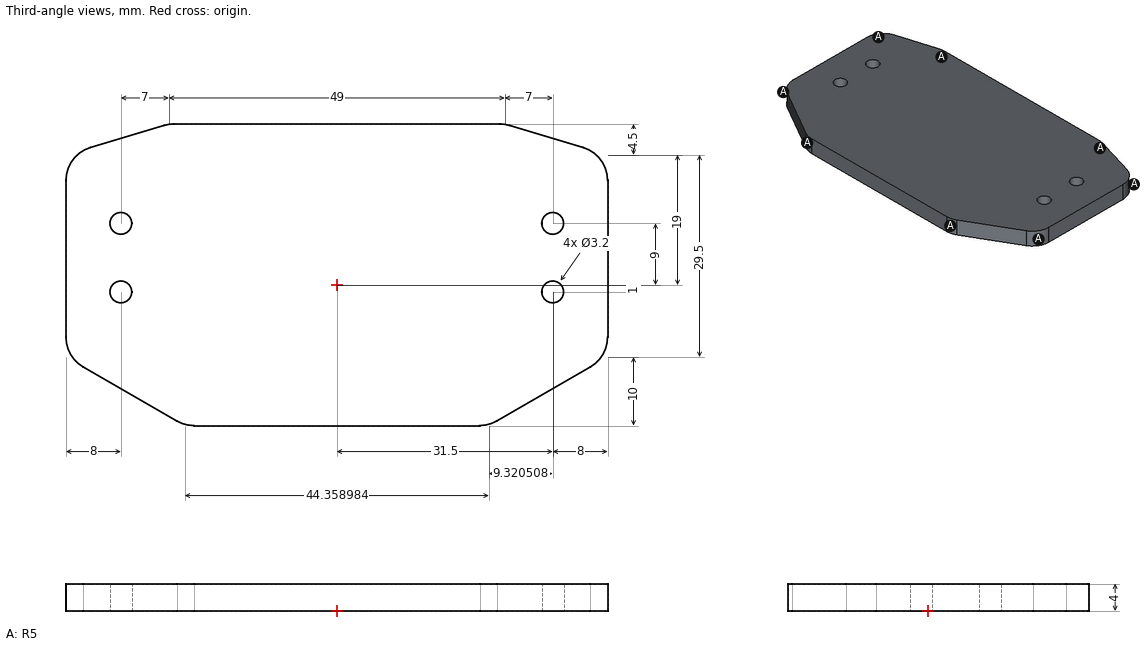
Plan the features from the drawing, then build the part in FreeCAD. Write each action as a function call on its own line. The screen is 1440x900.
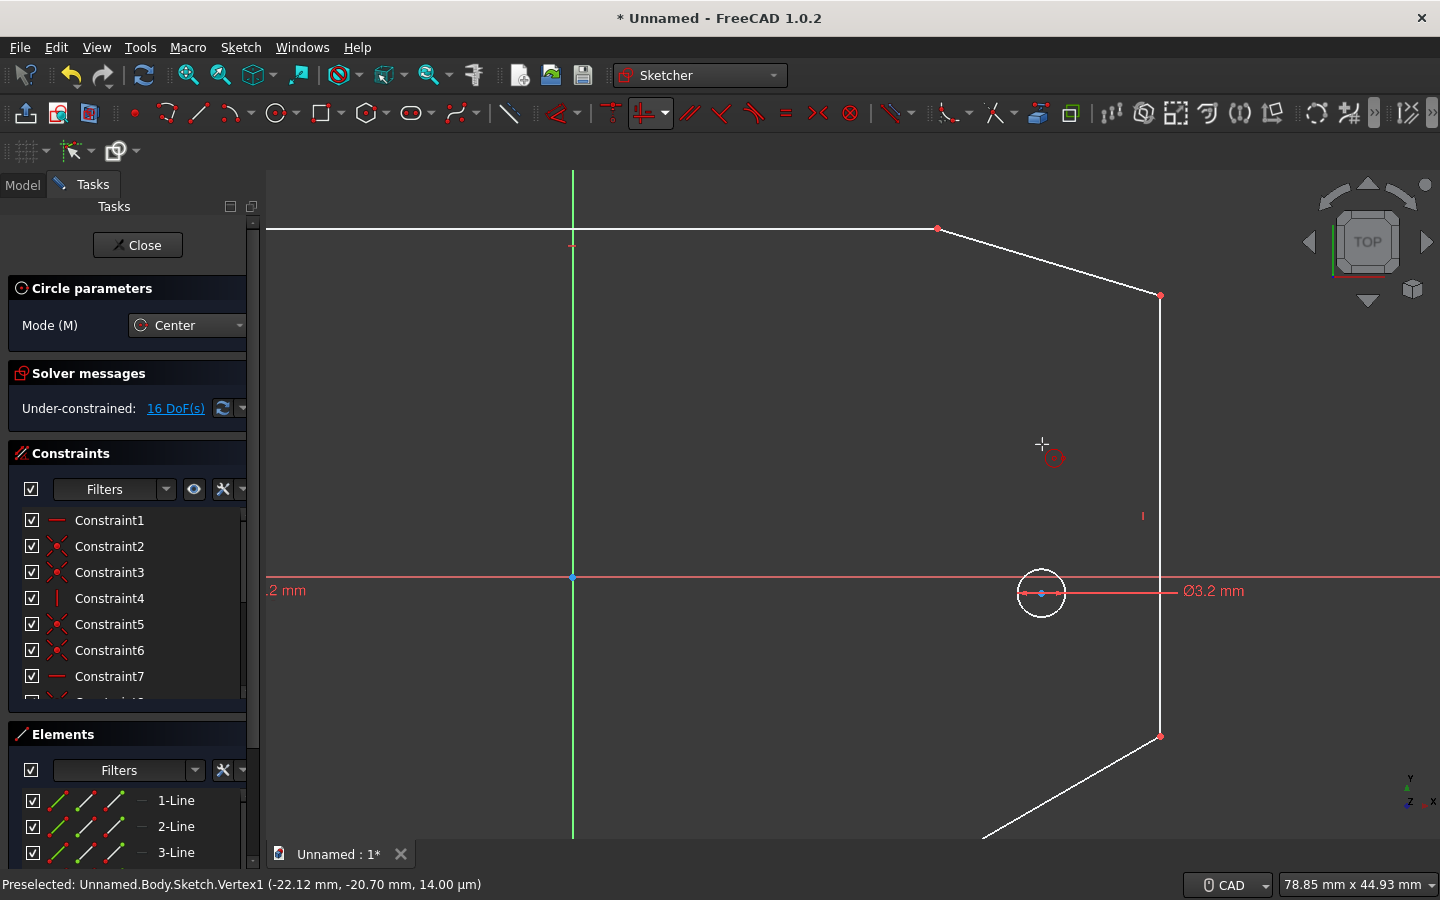
click(1042, 443)
move(1058, 426)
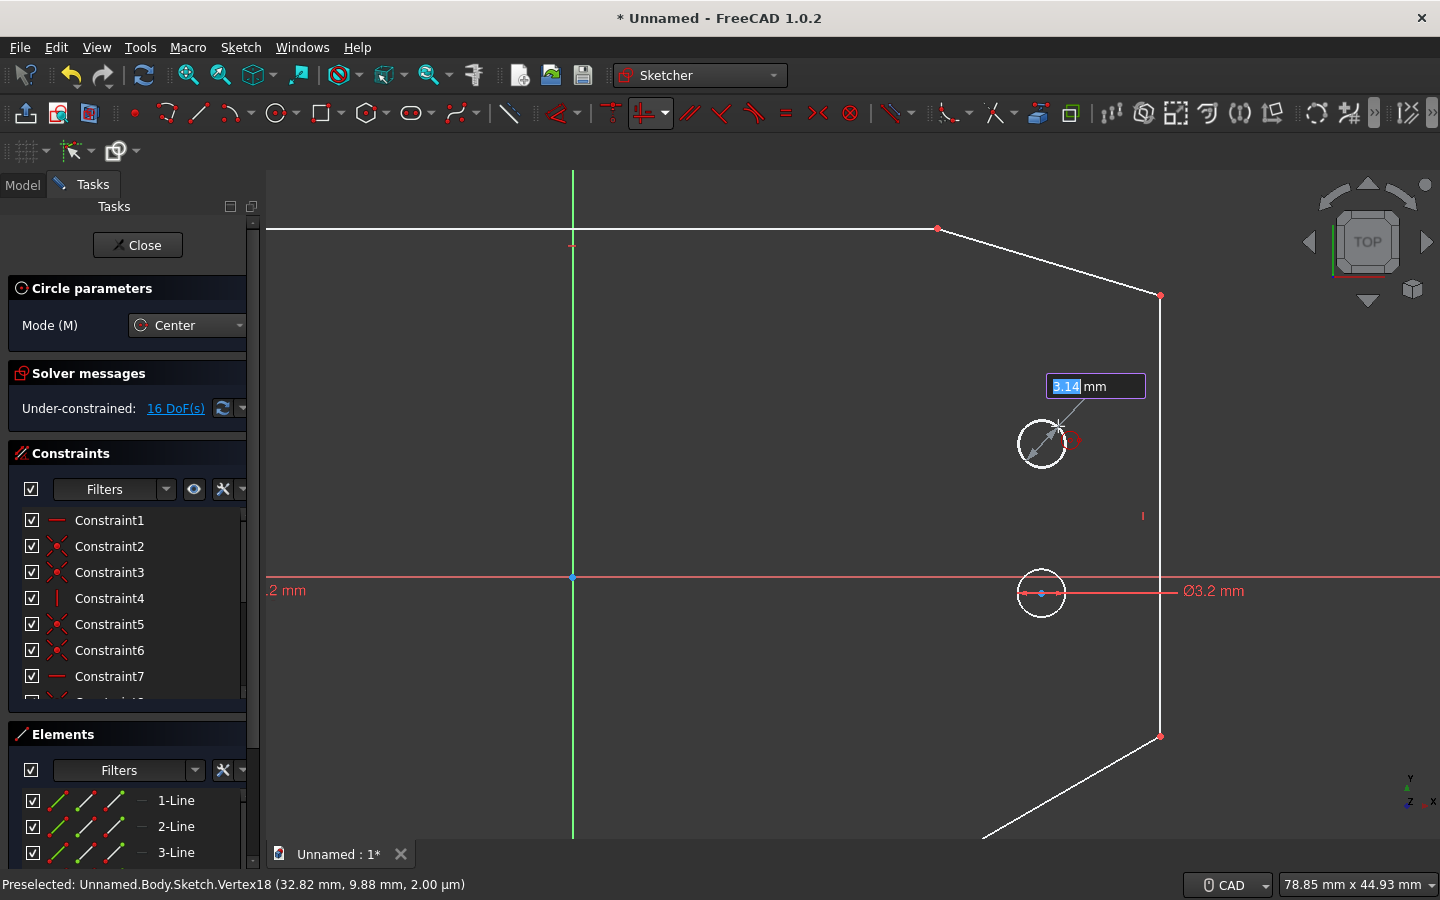
text(3.2)
key(Return)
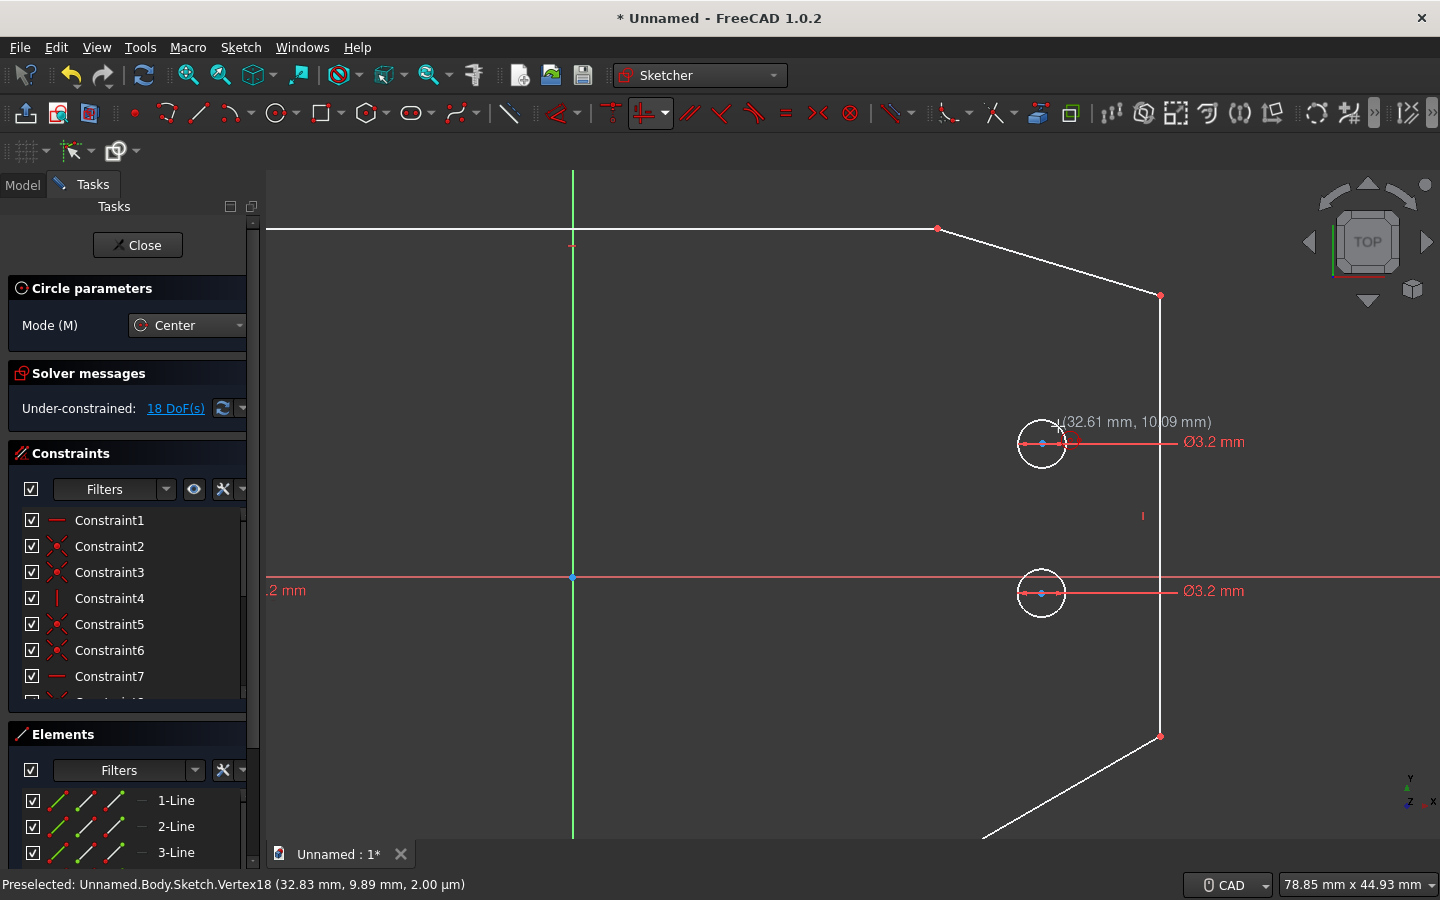
scroll(1042, 443, down, 3)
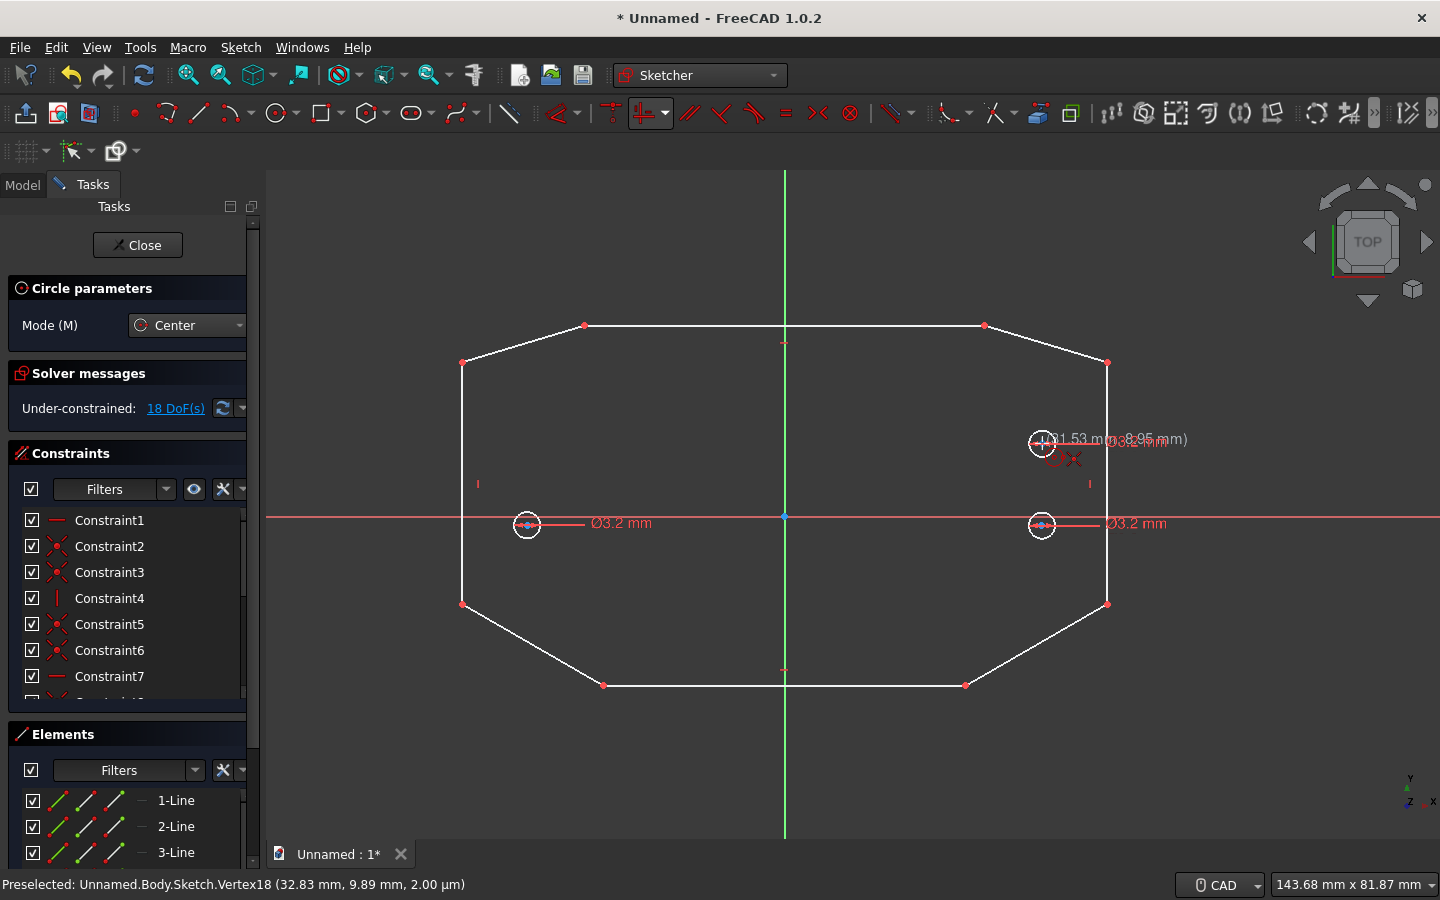
scroll(527, 443, up, 3)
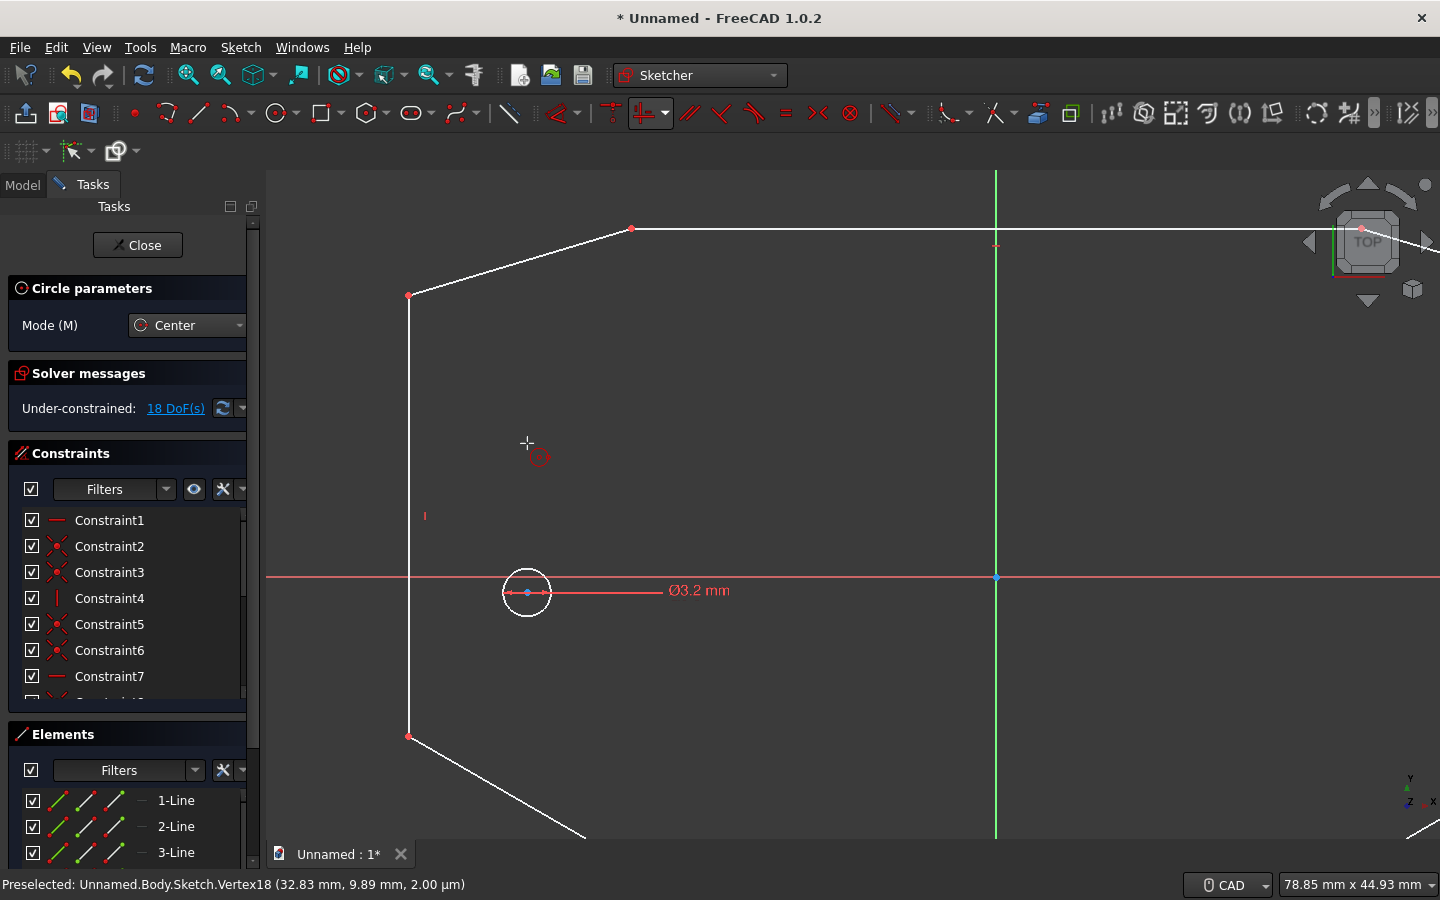
click(527, 443)
move(544, 426)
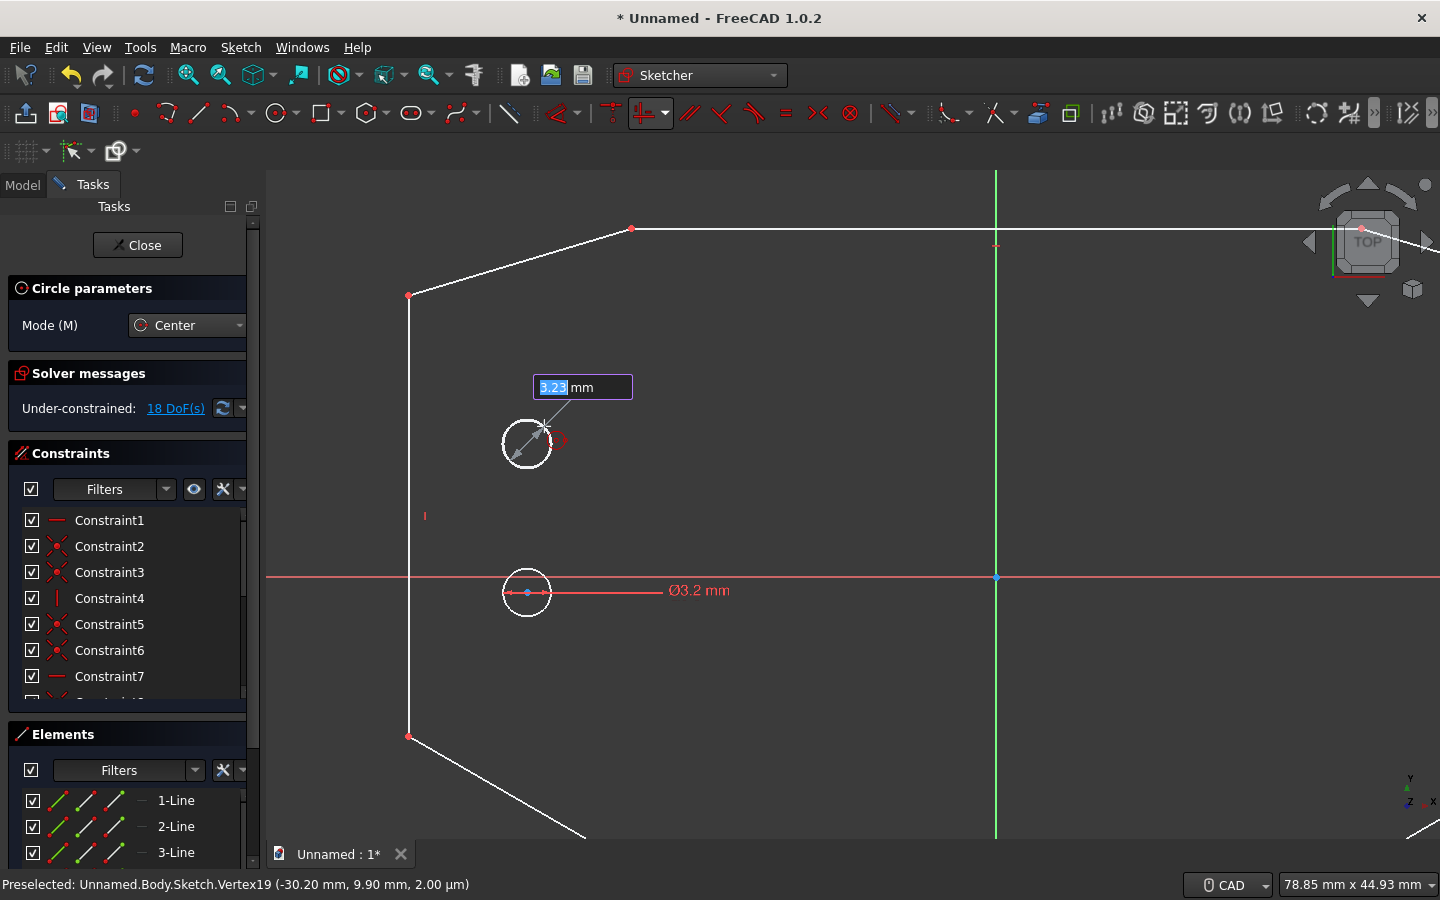
text(3.2)
key(Return)
key(Escape)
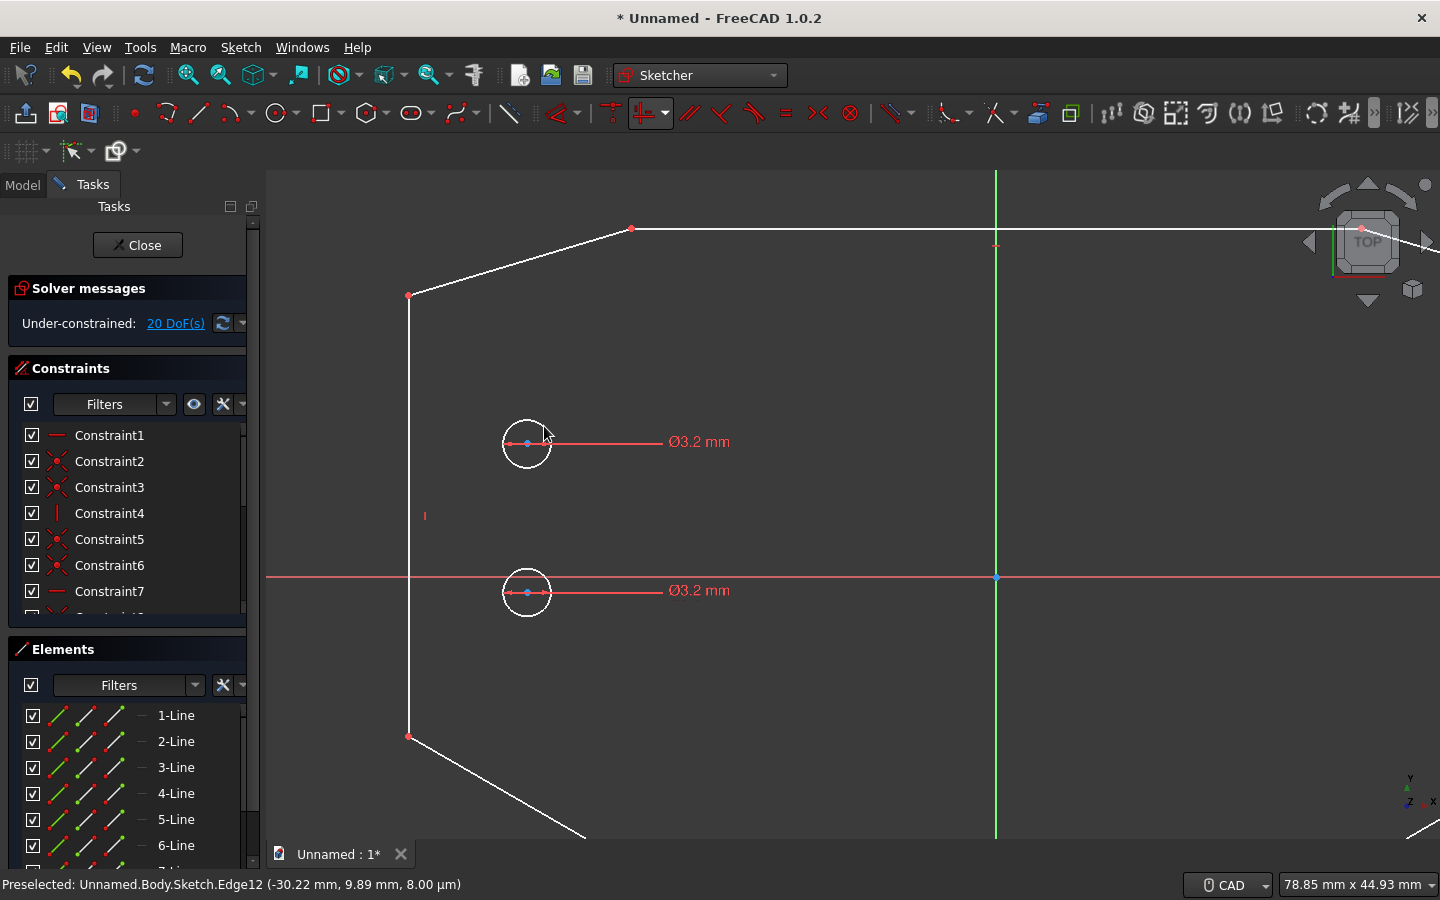
scroll(527, 443, down, 3)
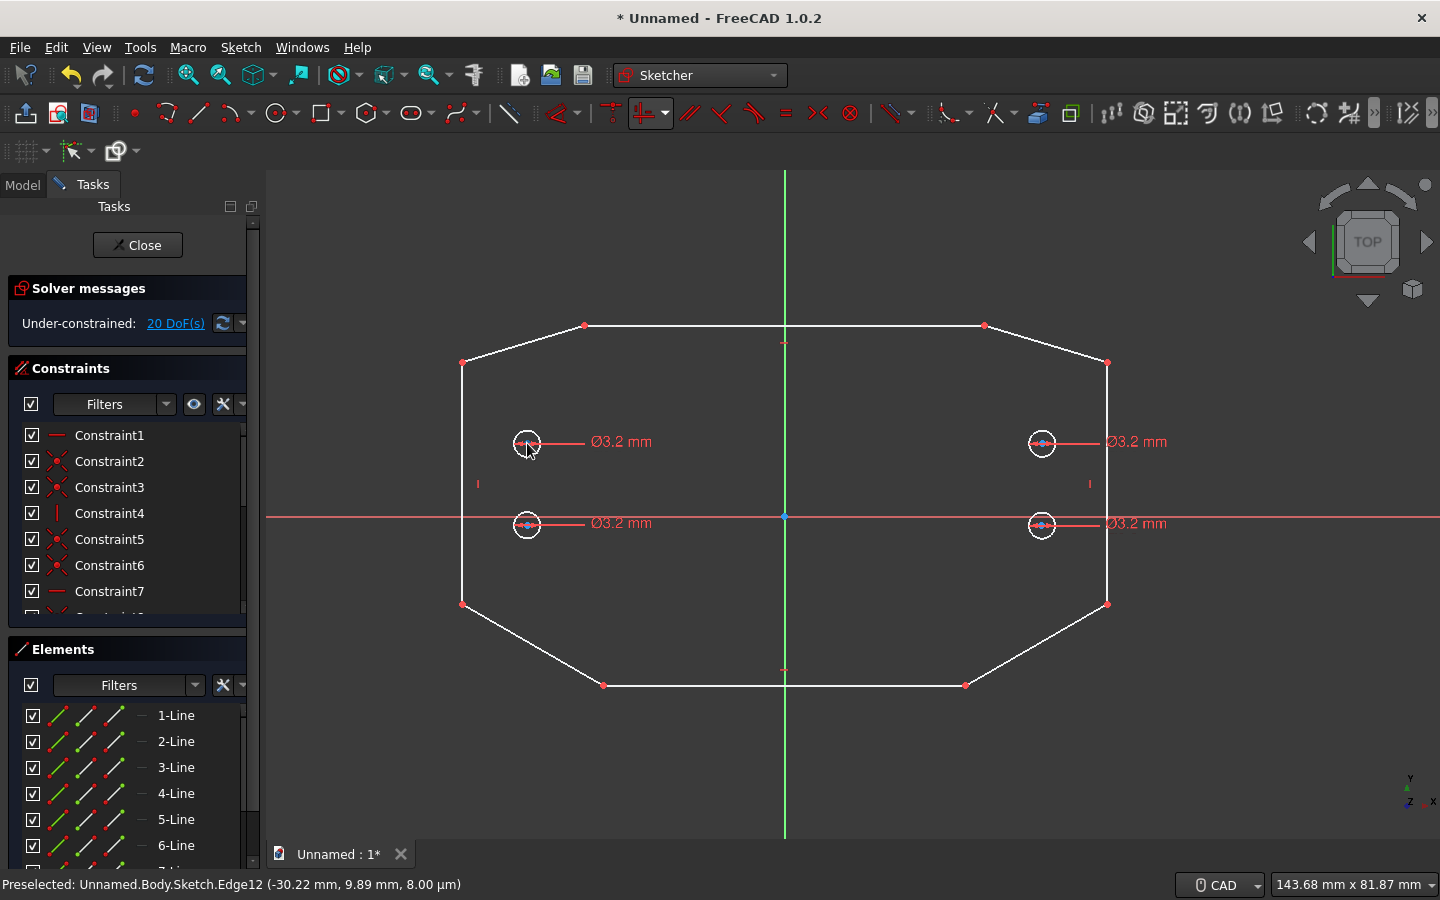
click(1042, 526)